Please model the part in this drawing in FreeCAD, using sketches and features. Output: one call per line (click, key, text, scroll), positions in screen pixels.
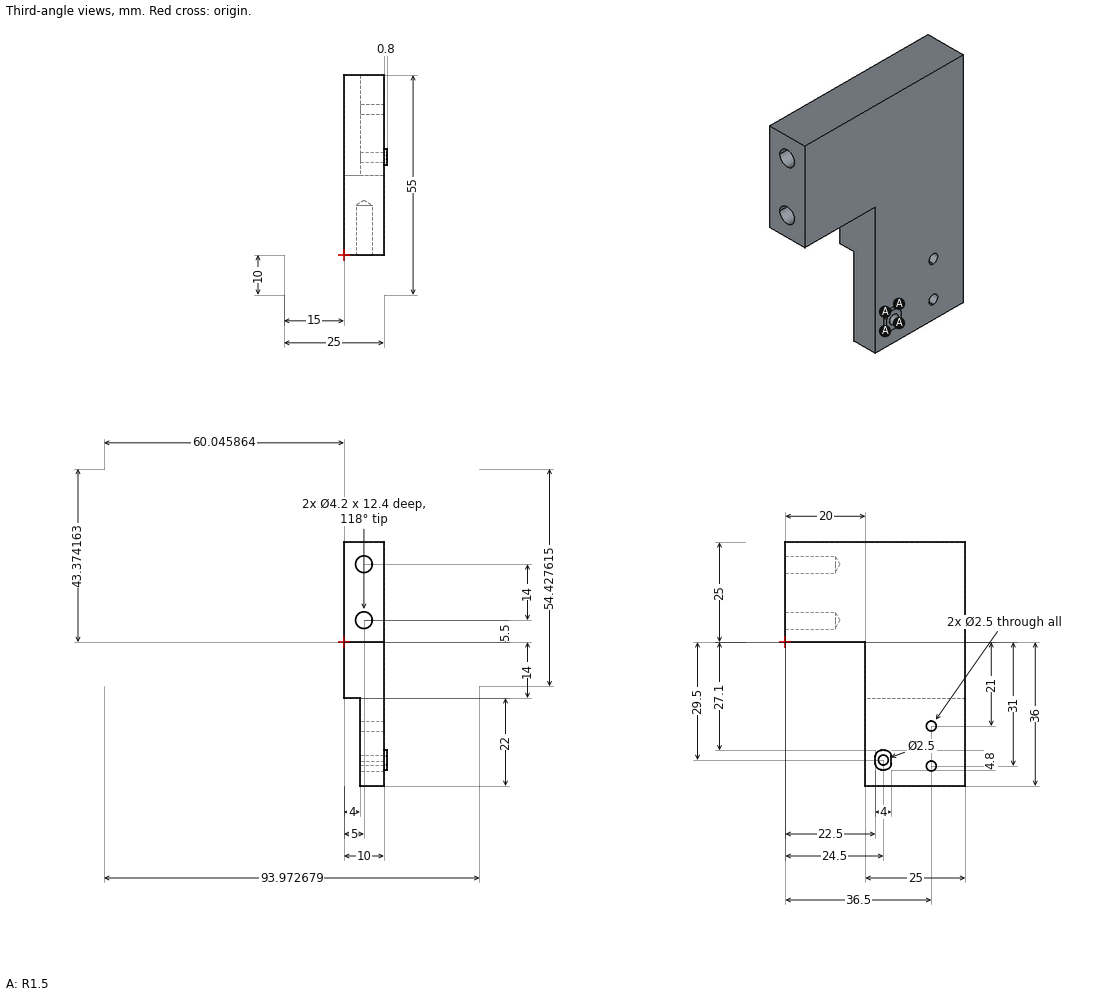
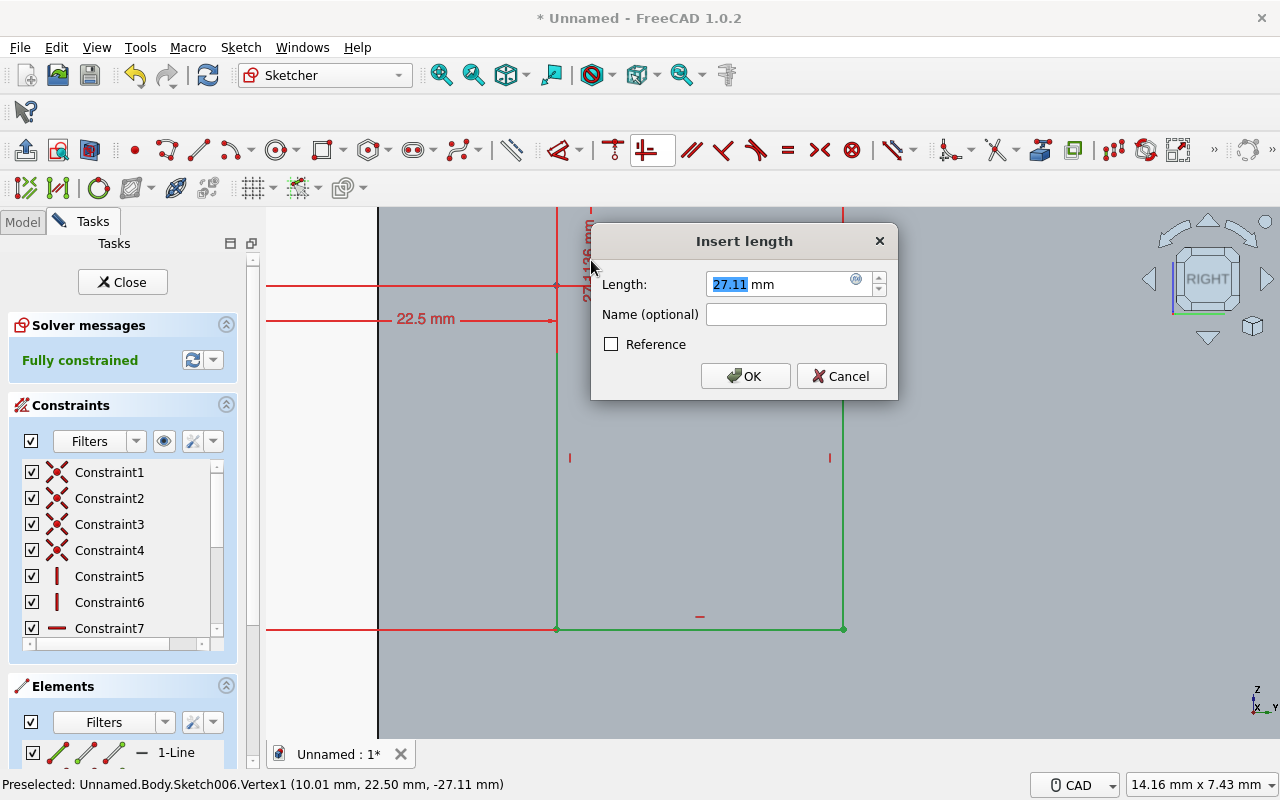
text(27.1)
key(Return)
key(Escape)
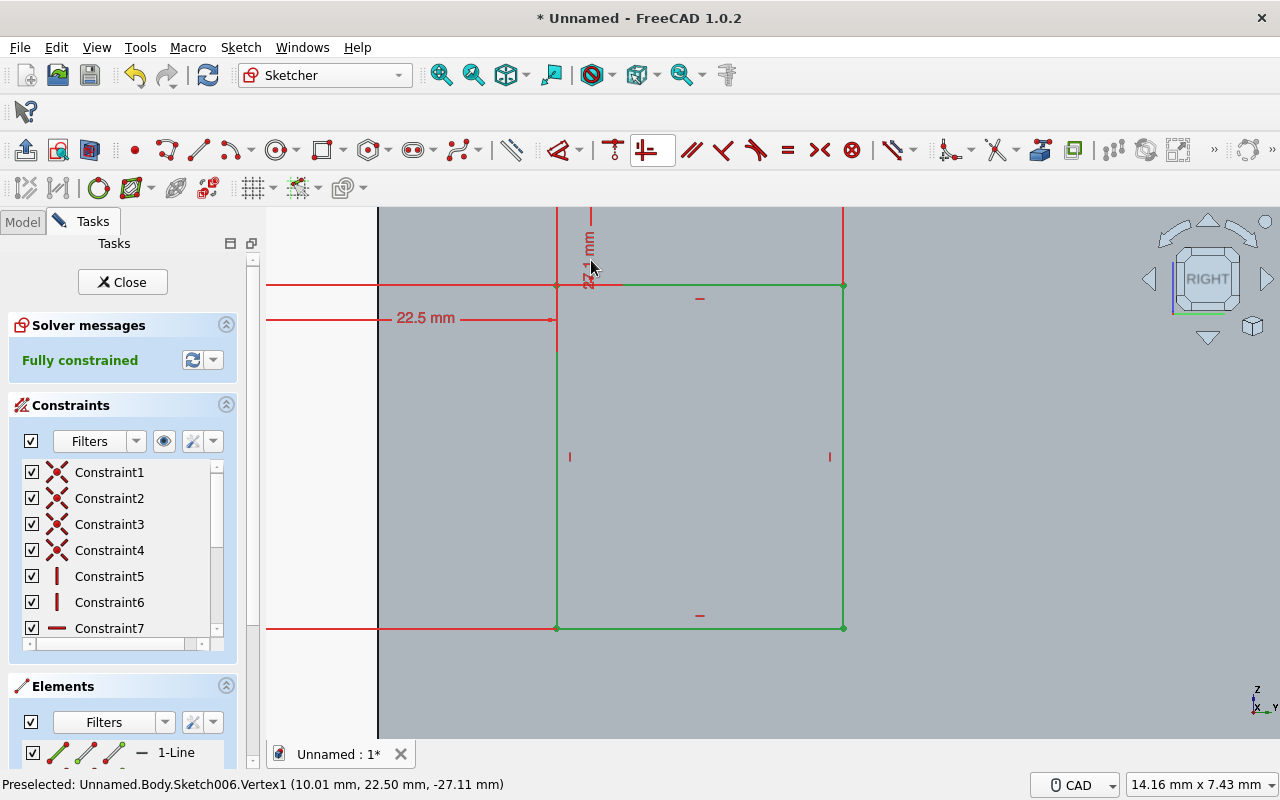
click(123, 282)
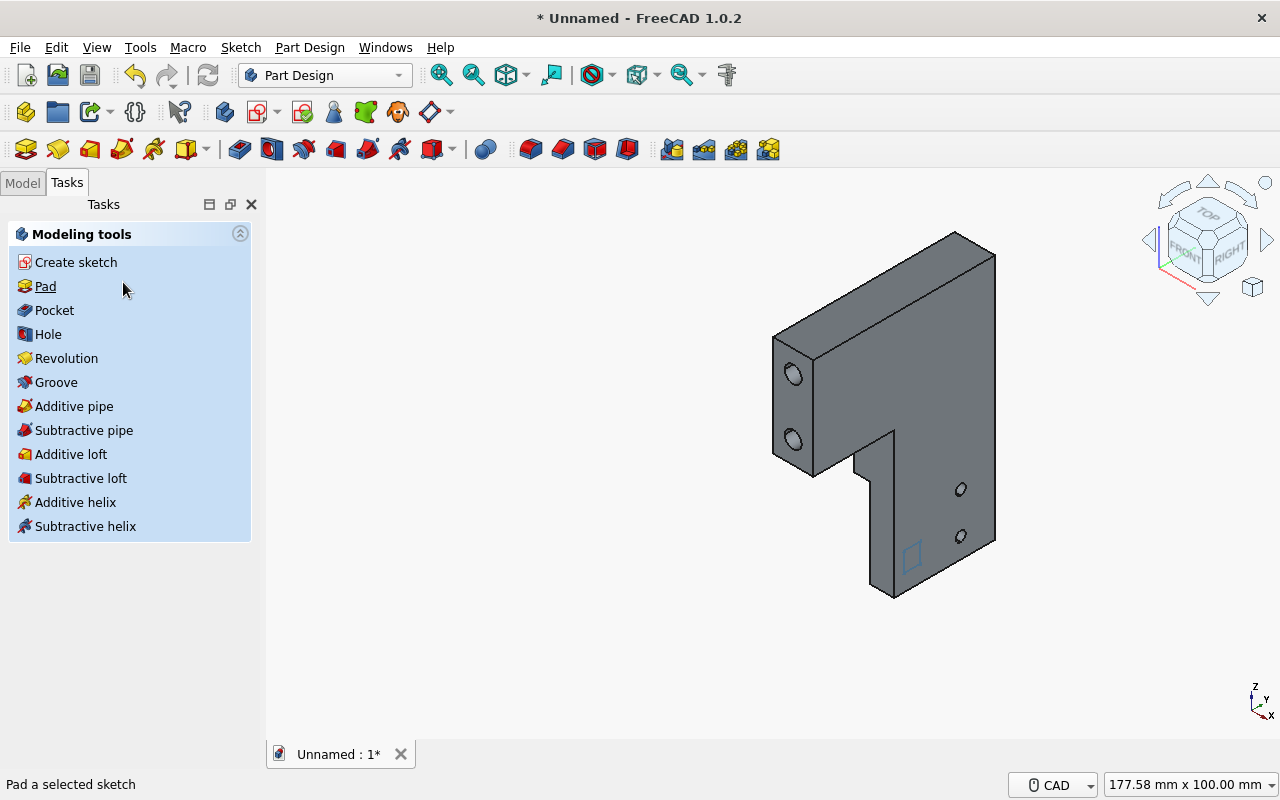
click(26, 150)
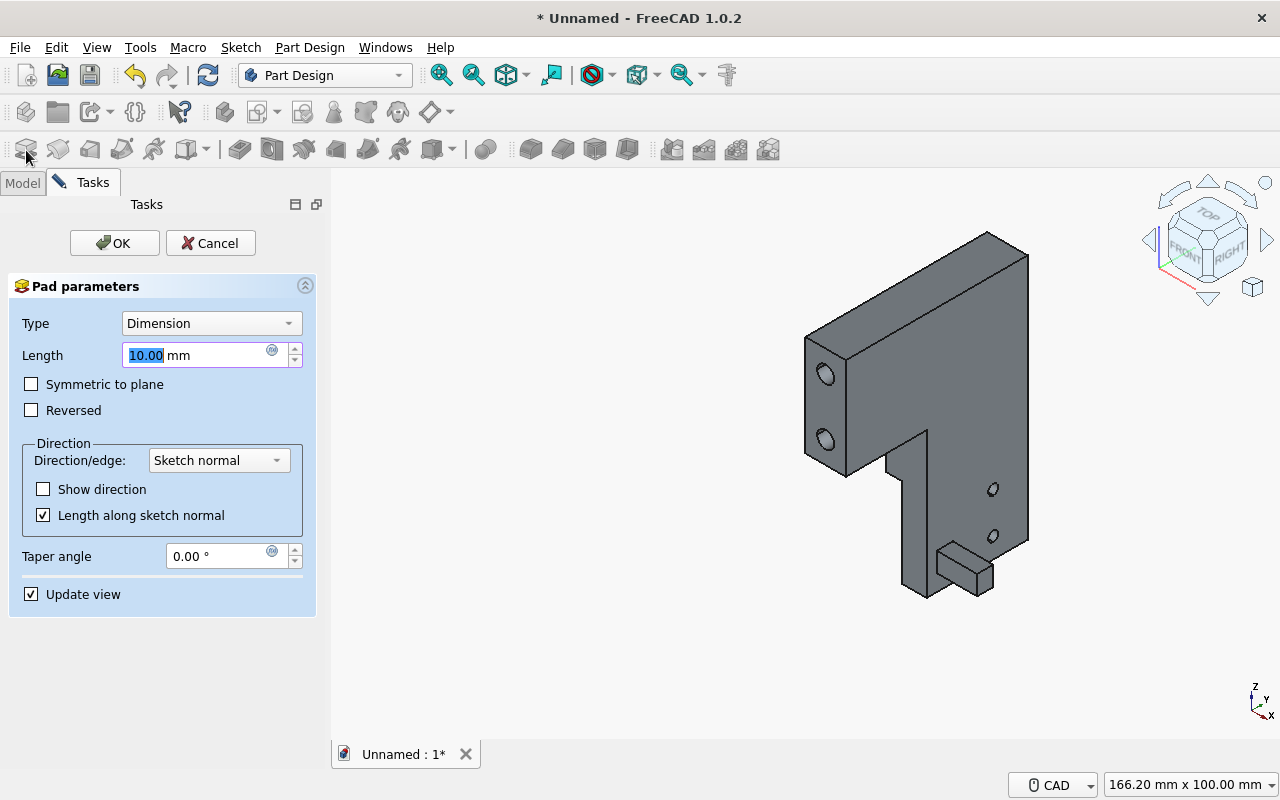
text(0.8)
key(Tab)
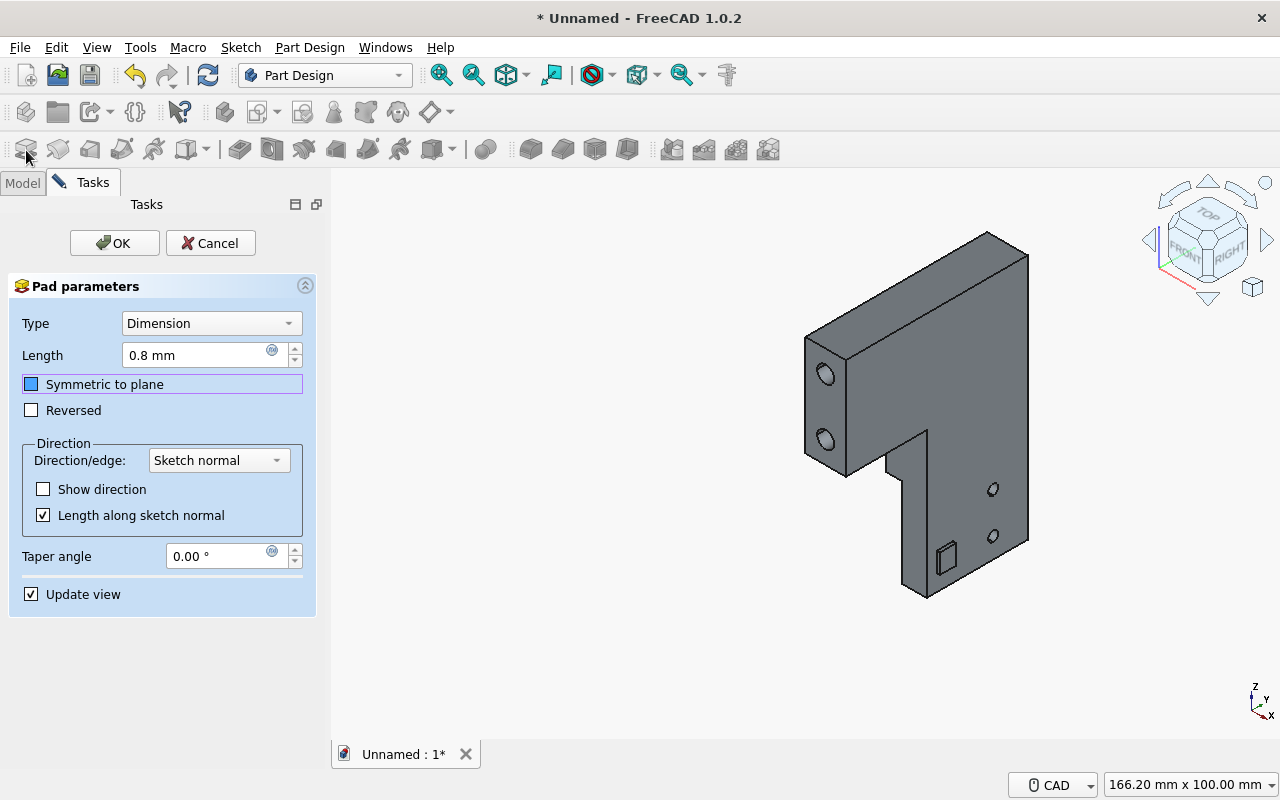
click(115, 243)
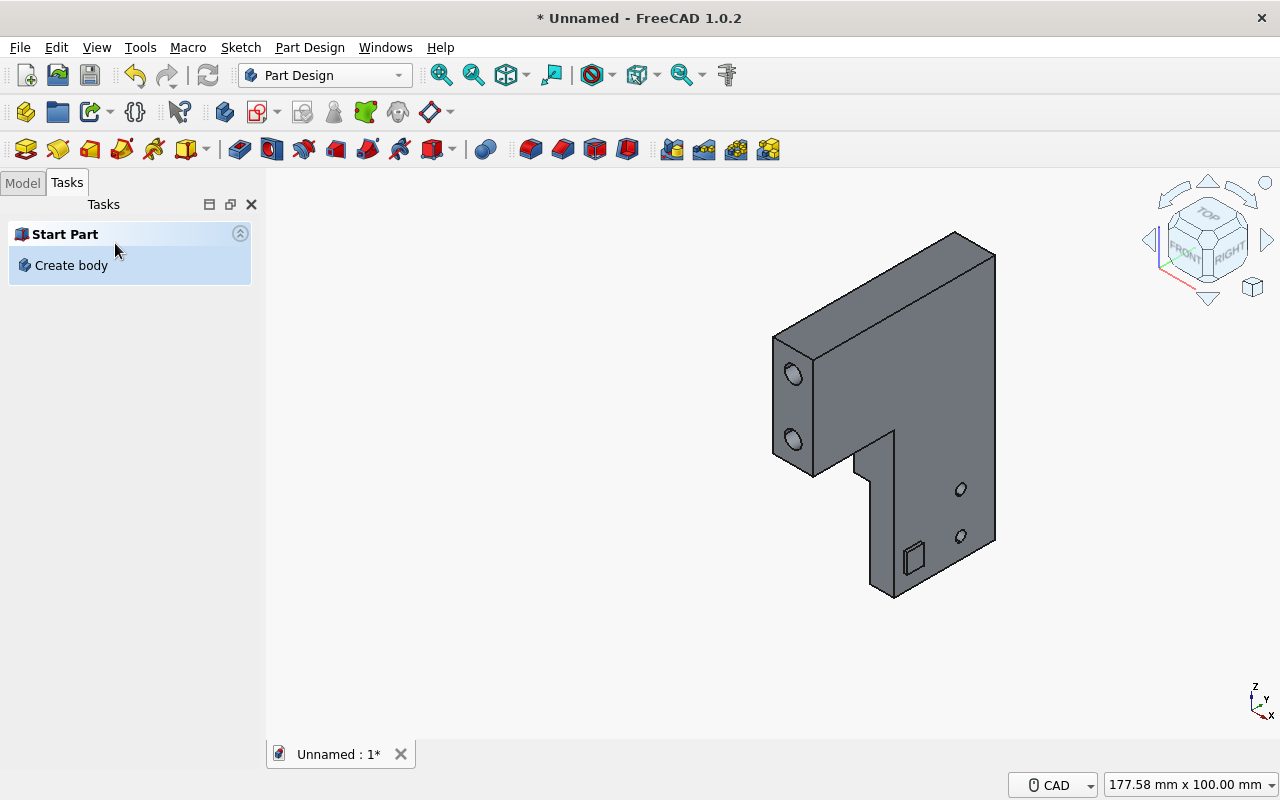
key(6)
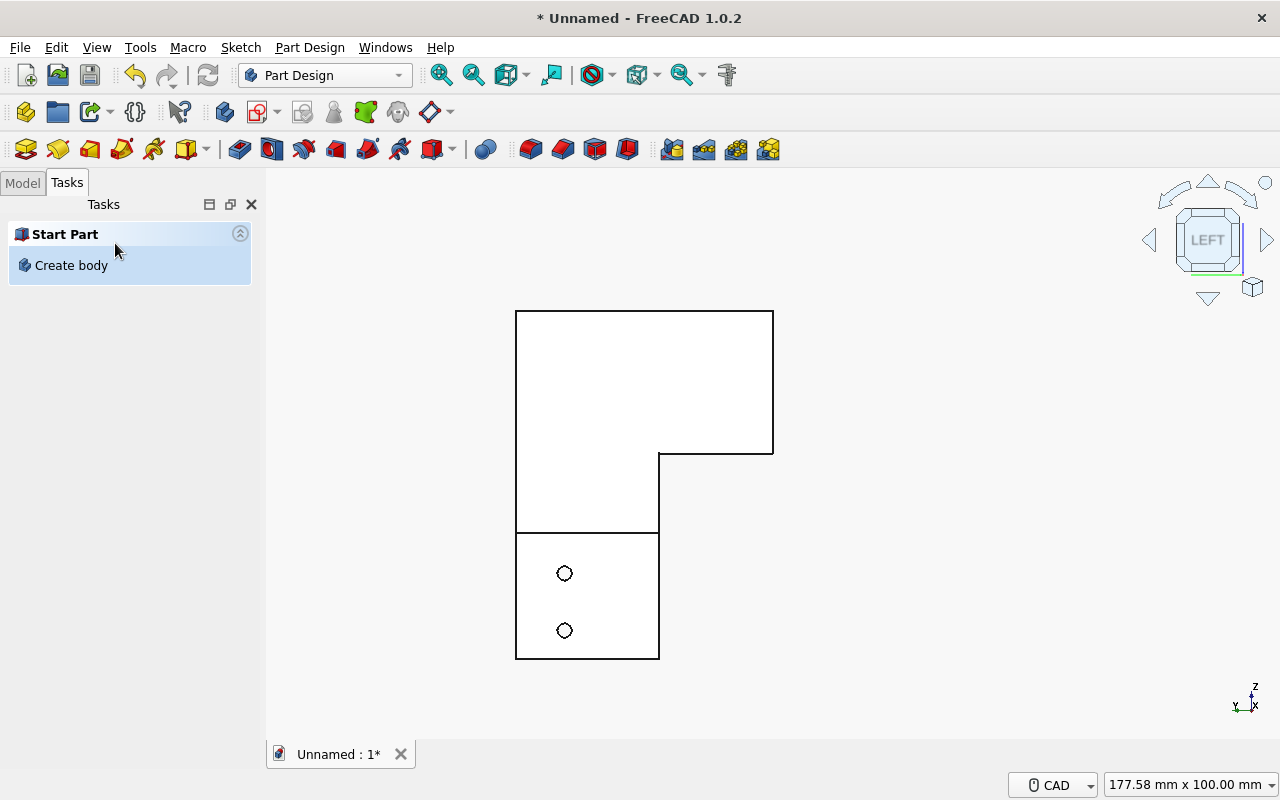
click(608, 389)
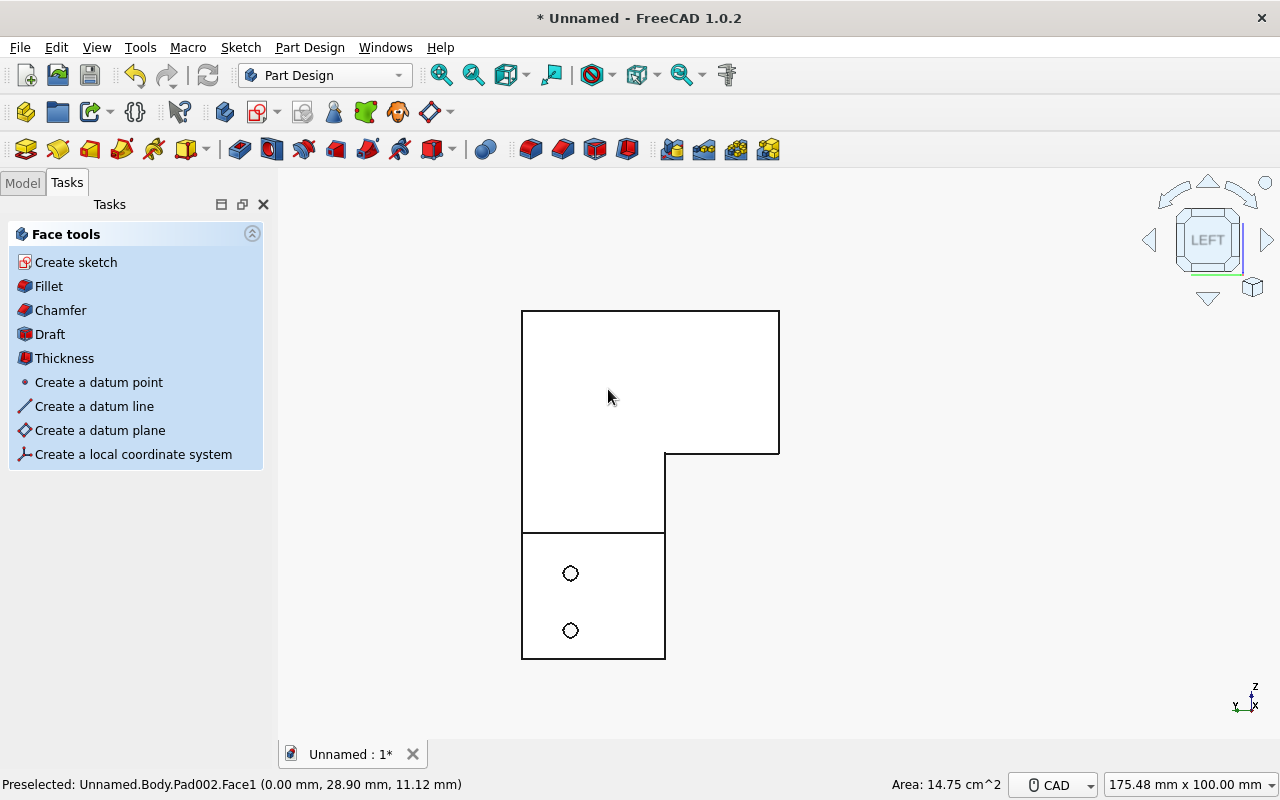
click(258, 112)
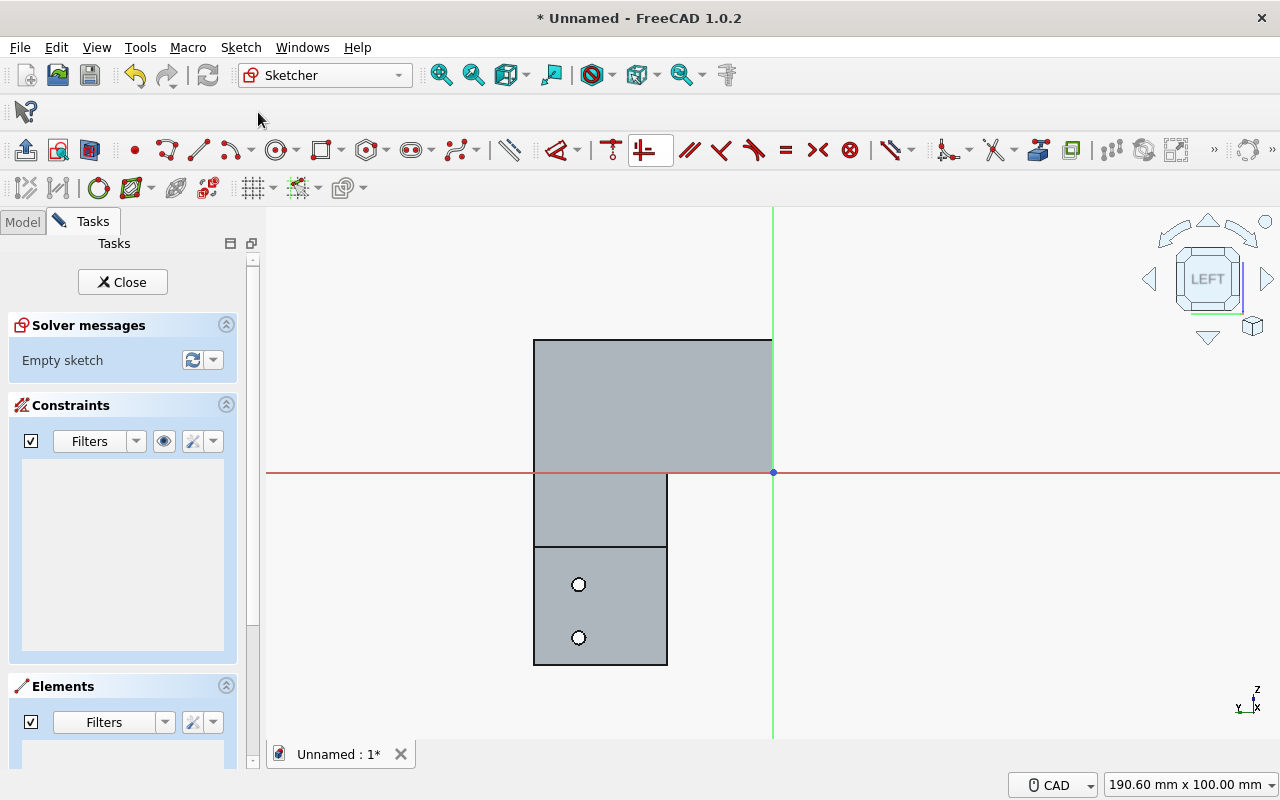
scroll(639, 638, up, 15)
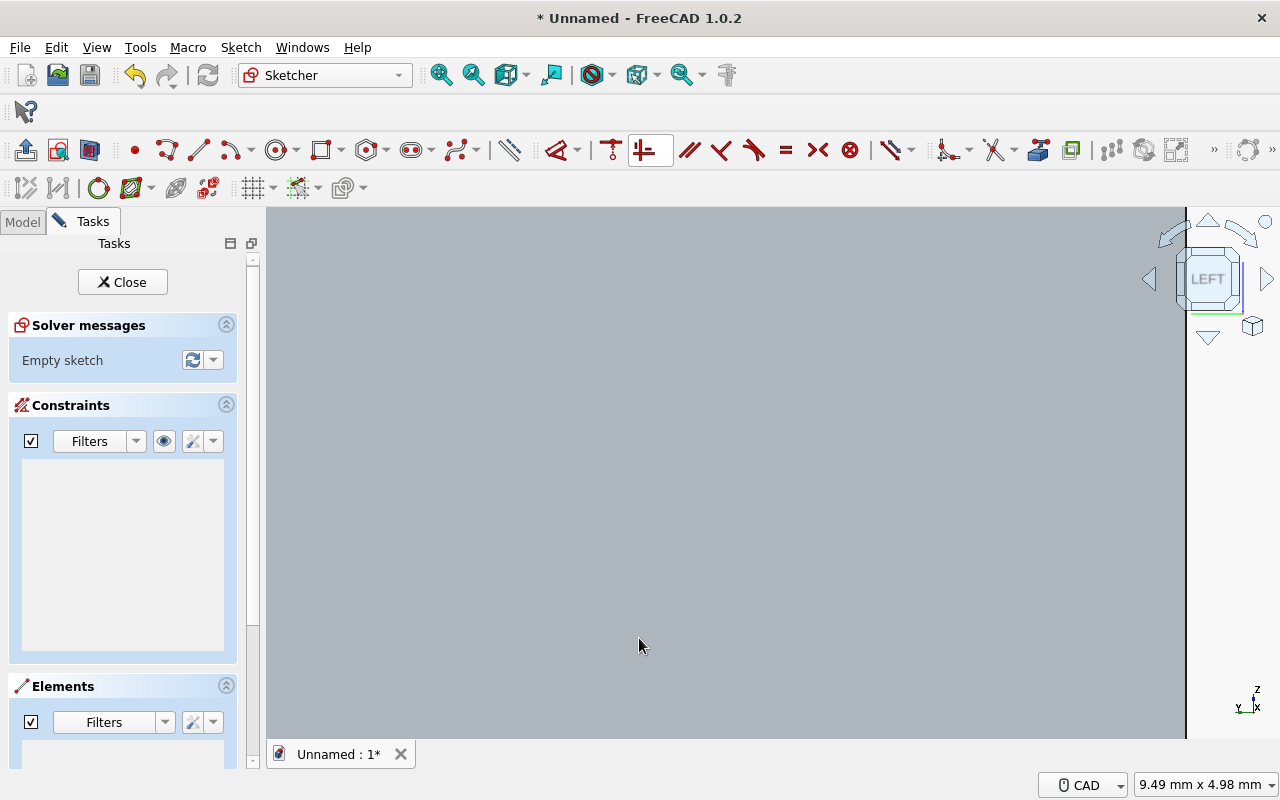
key(g)
key(c)